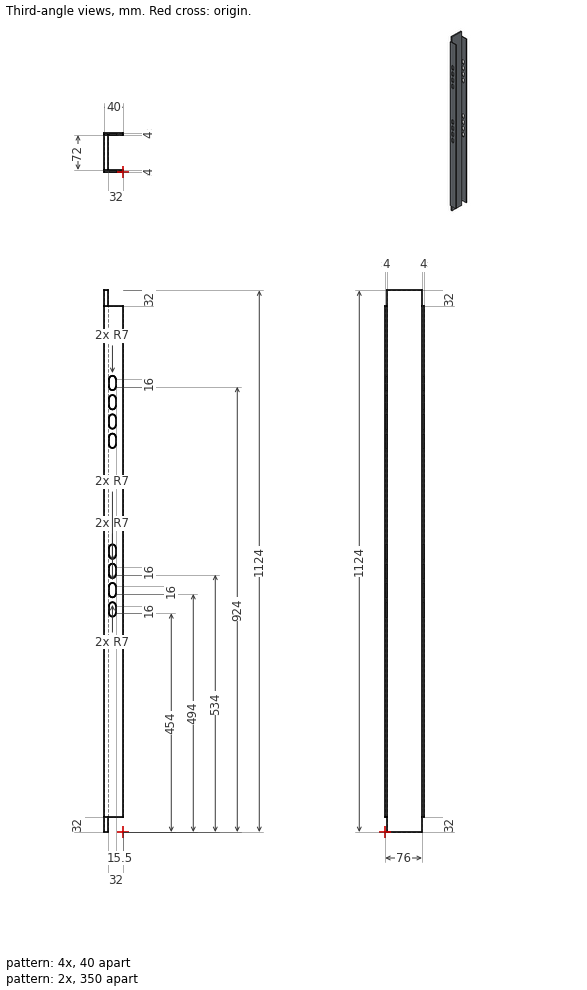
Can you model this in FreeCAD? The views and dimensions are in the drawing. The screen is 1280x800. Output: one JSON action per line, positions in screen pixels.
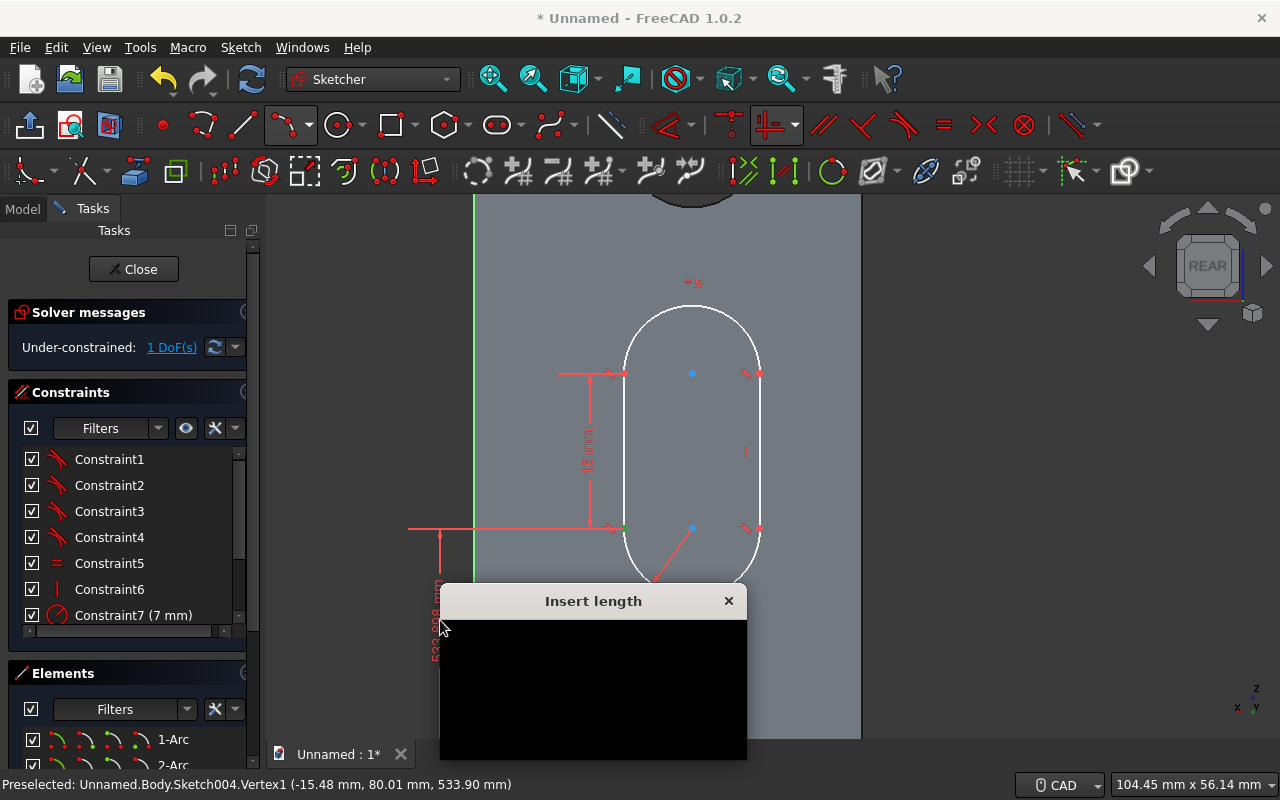
{"action": "type", "text": "534"}
{"action": "key", "text": "Return"}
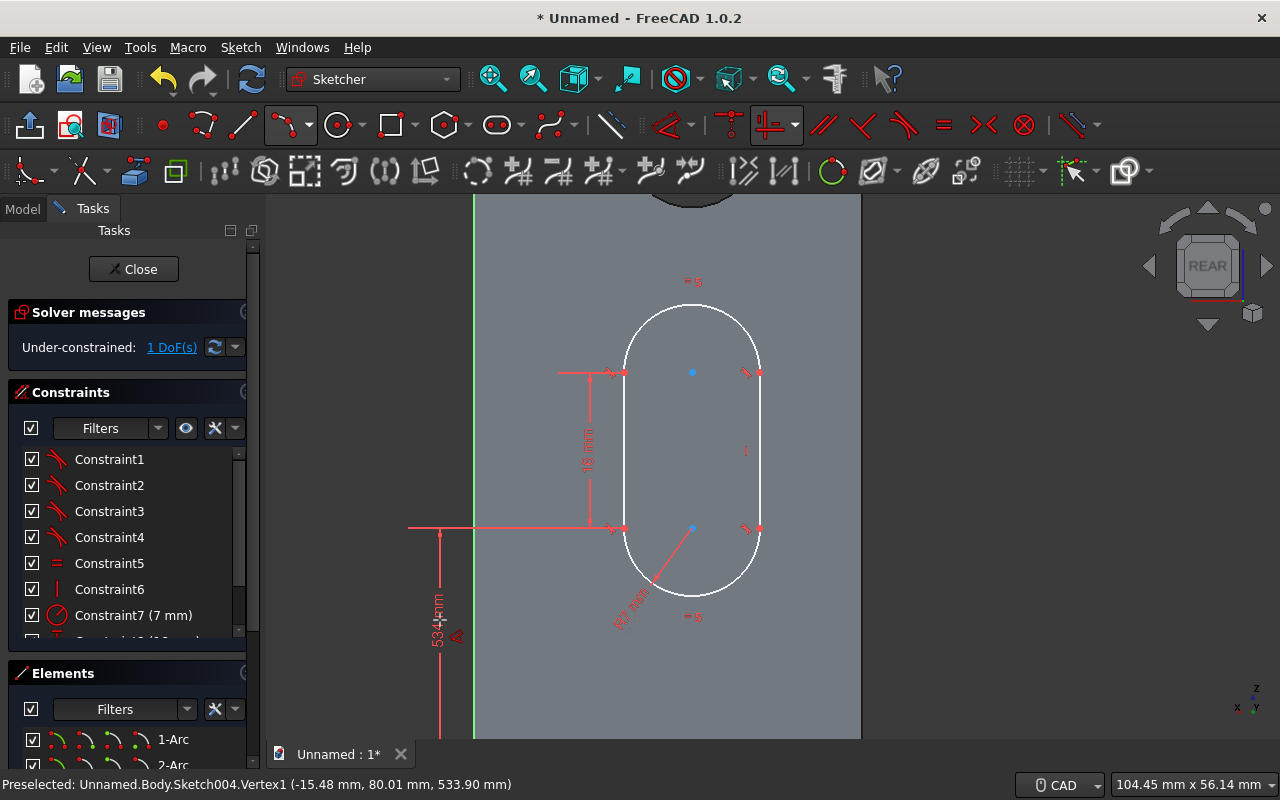
{"action": "left_click", "coordinate": [624, 528]}
{"action": "left_click", "coordinate": [549, 494]}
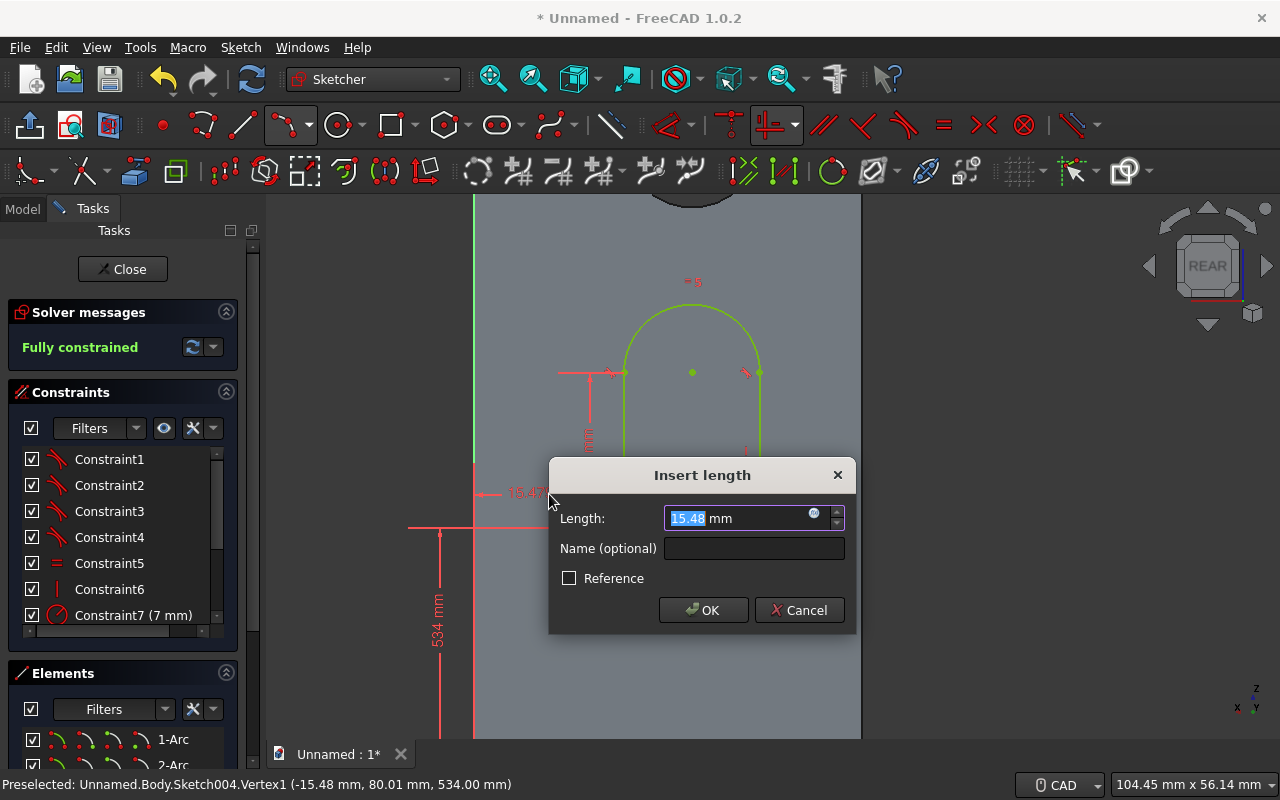
{"action": "type", "text": "15.5"}
{"action": "key", "text": "Return"}
{"action": "key", "text": "Escape"}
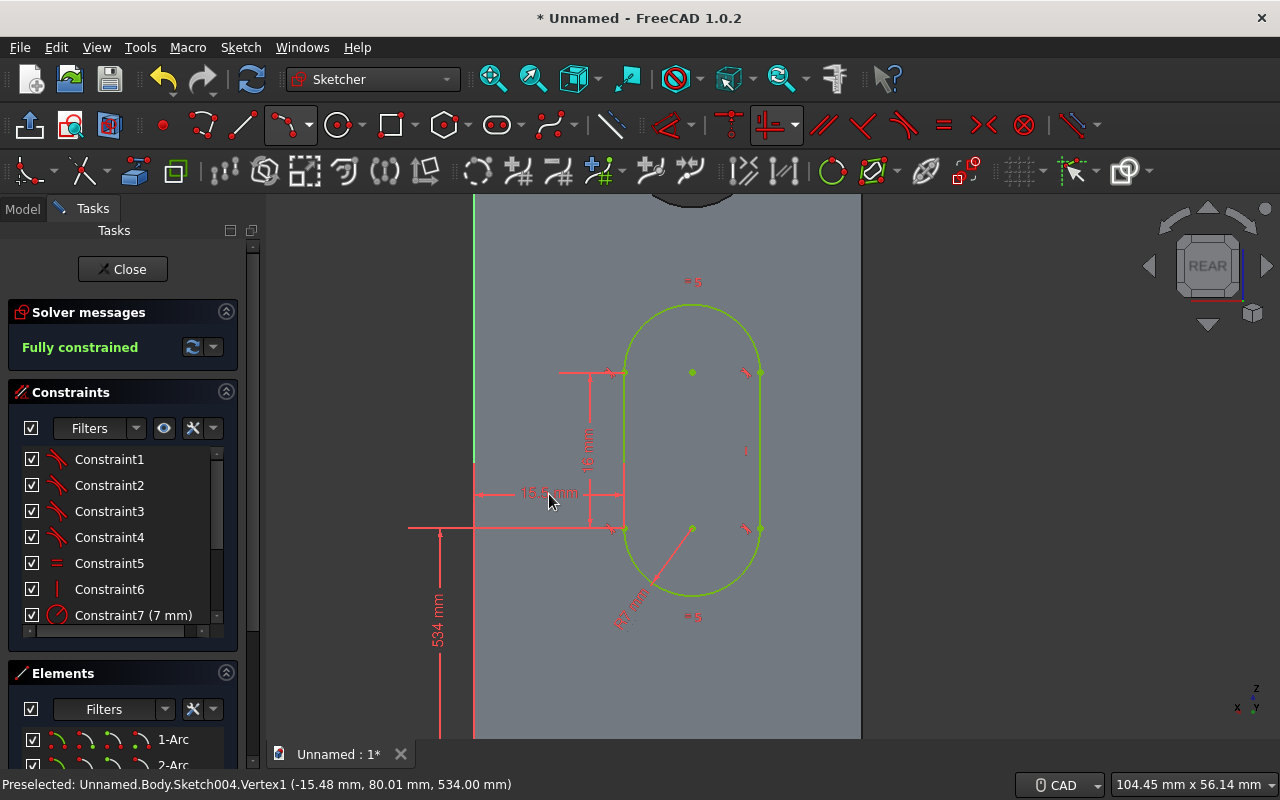
{"action": "left_click", "coordinate": [123, 269]}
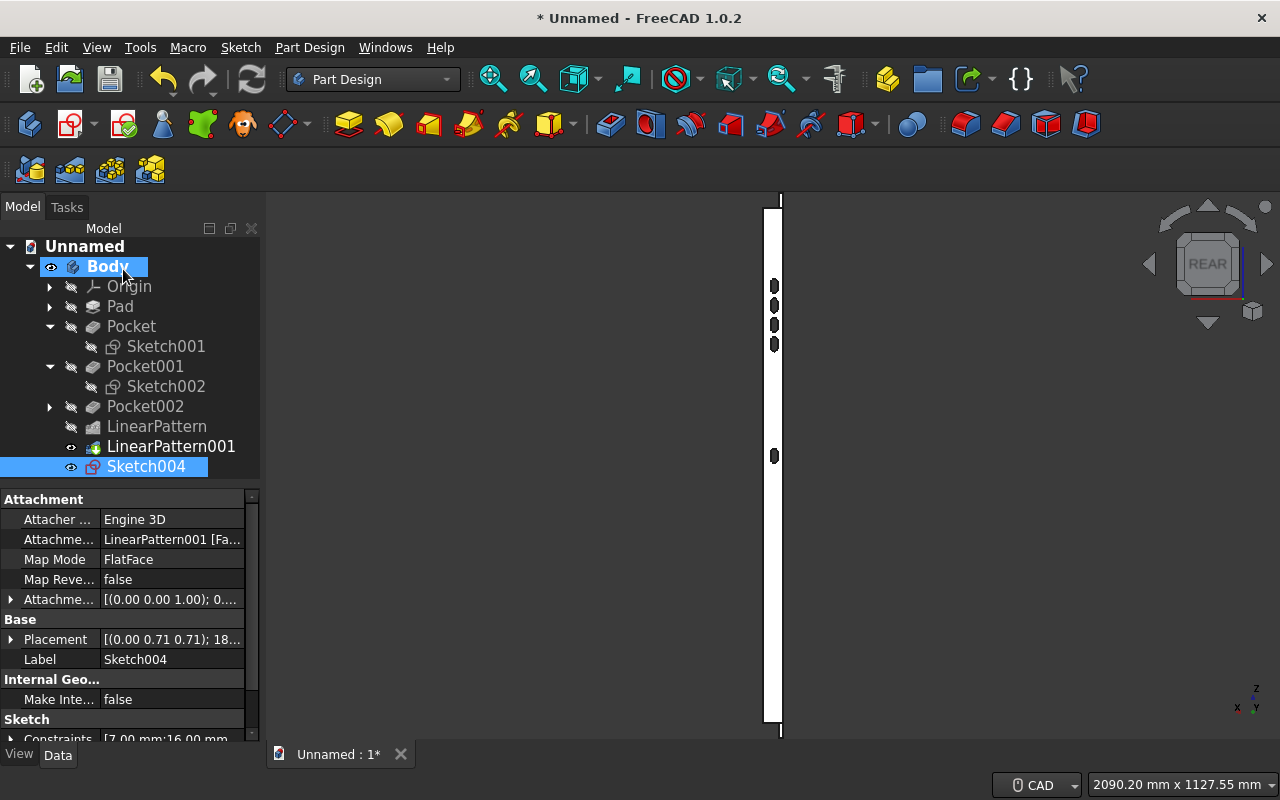
{"action": "left_click", "coordinate": [612, 124]}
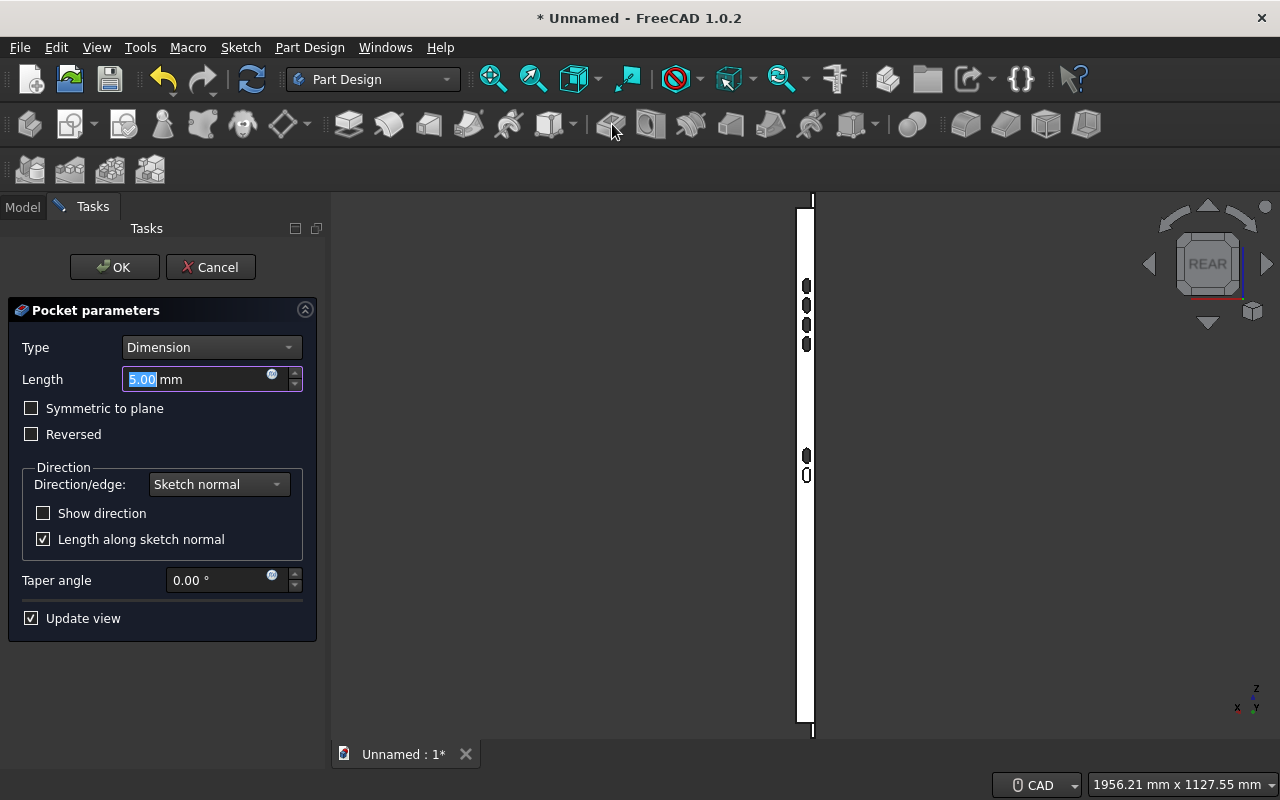
{"action": "left_click", "coordinate": [212, 348]}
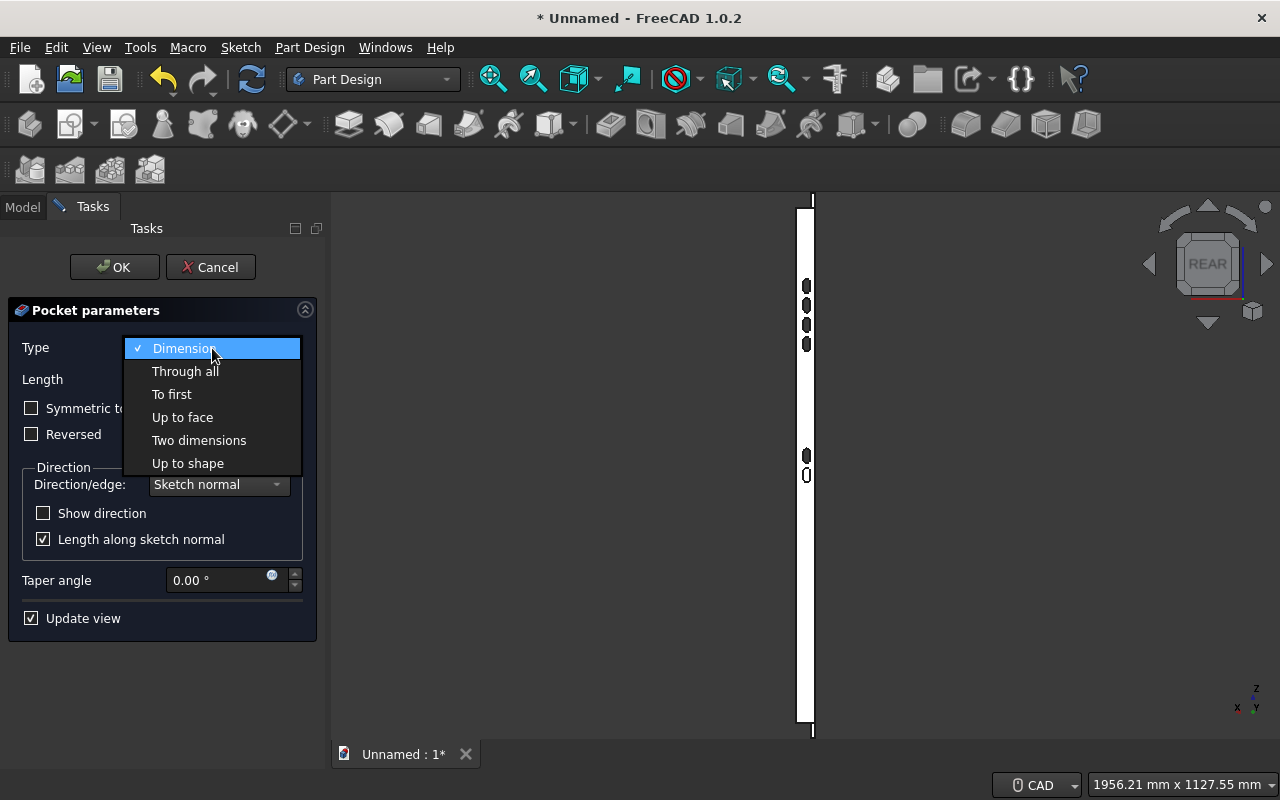
{"action": "left_click", "coordinate": [212, 372]}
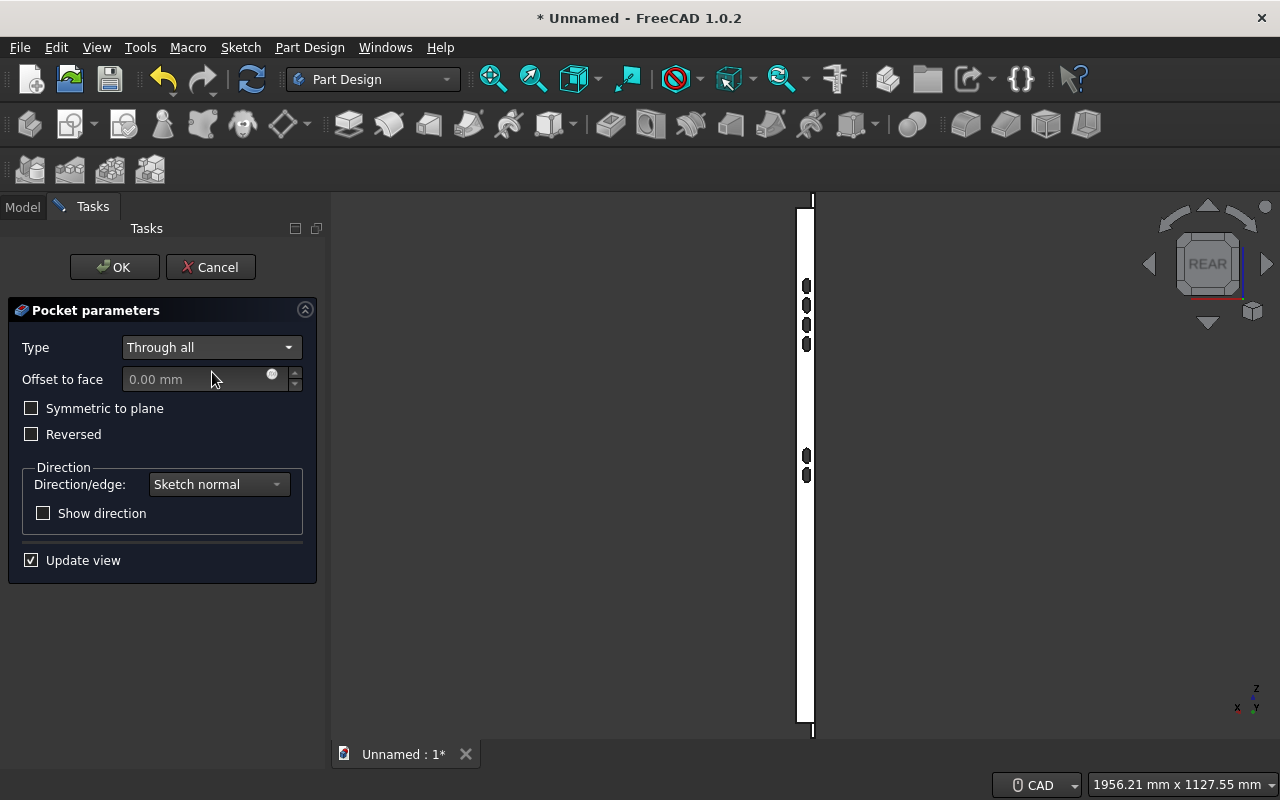
{"action": "left_click", "coordinate": [115, 267]}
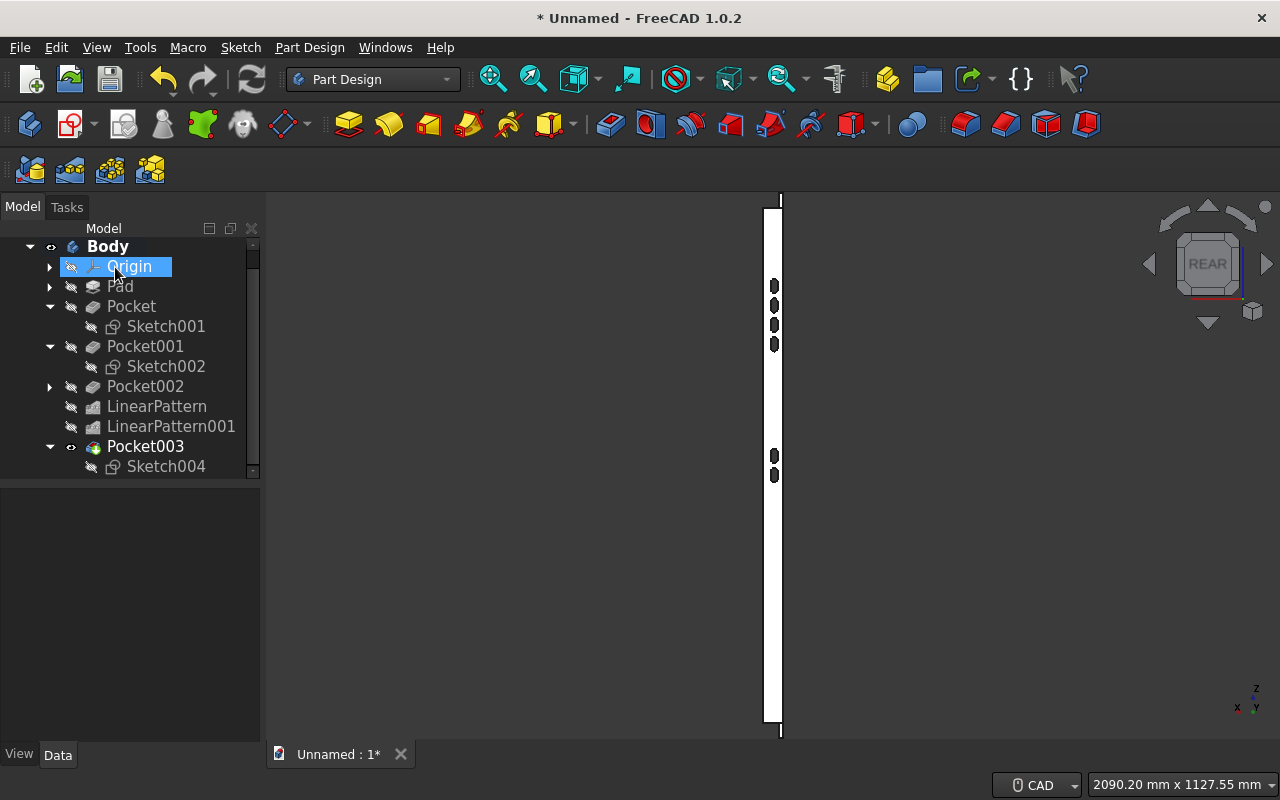
{"action": "left_click", "coordinate": [773, 244]}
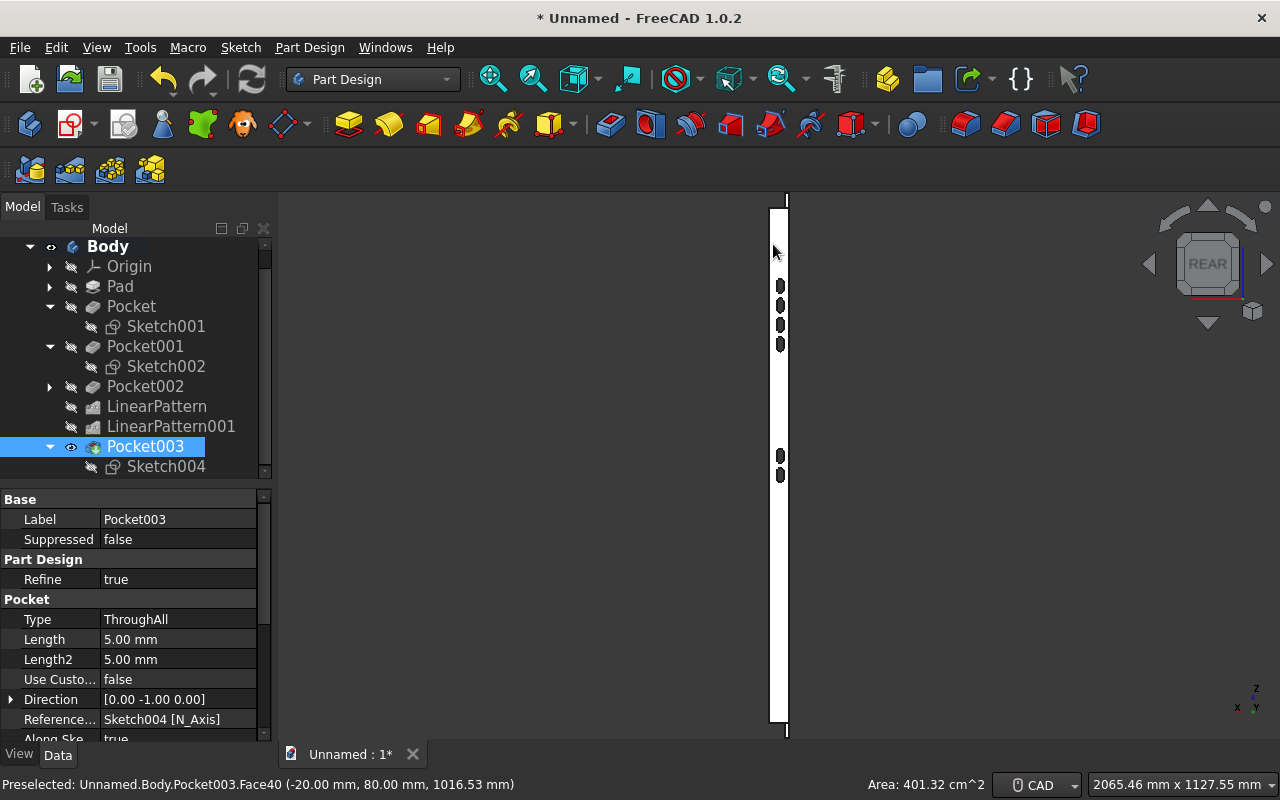
{"action": "left_click", "coordinate": [70, 124]}